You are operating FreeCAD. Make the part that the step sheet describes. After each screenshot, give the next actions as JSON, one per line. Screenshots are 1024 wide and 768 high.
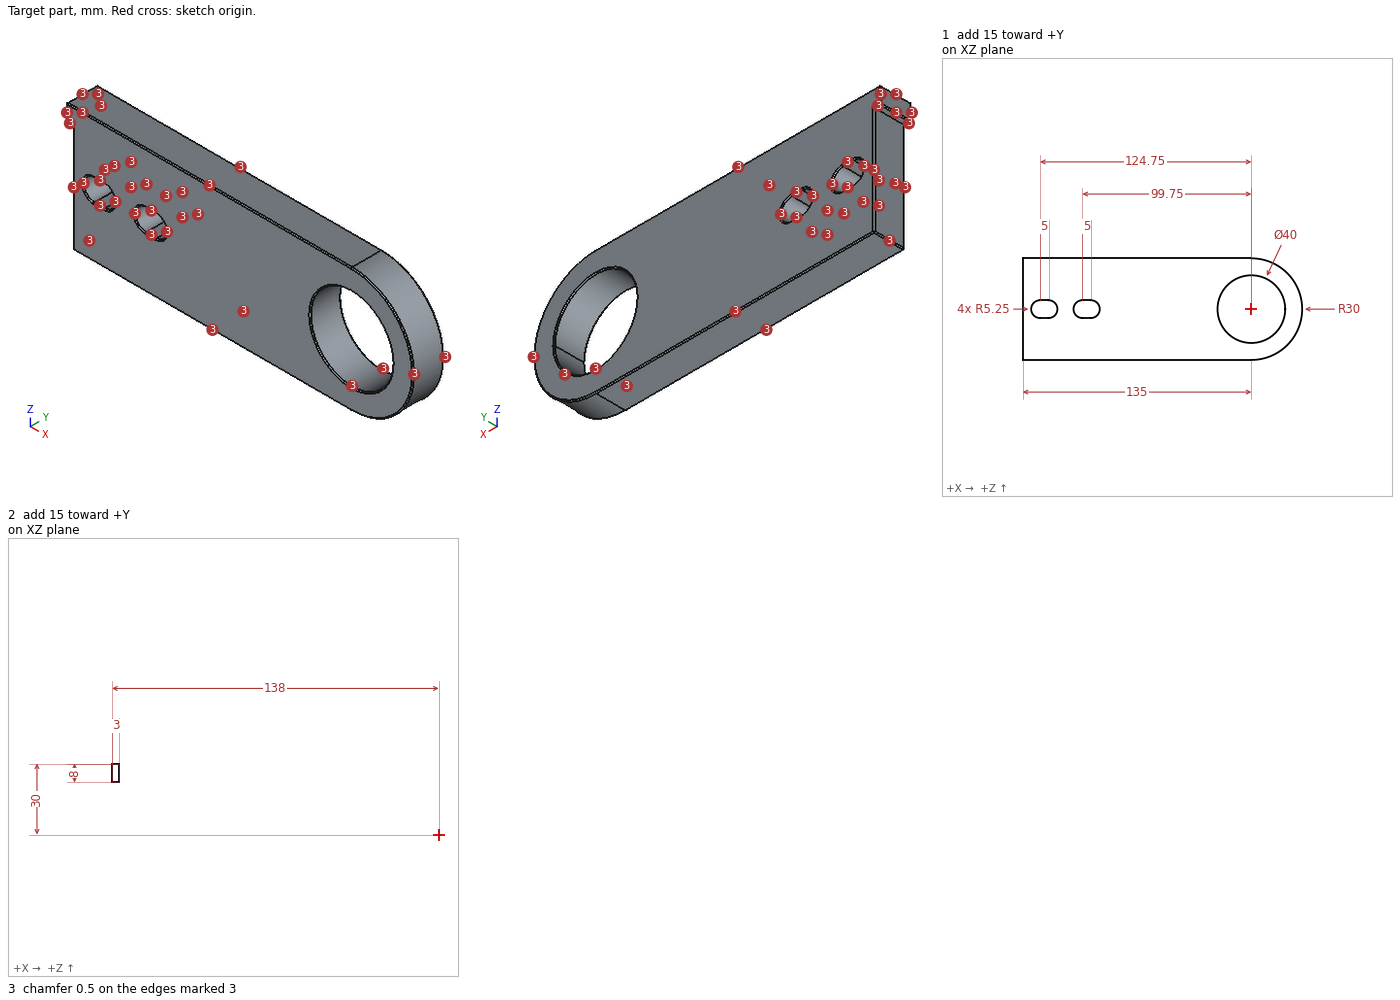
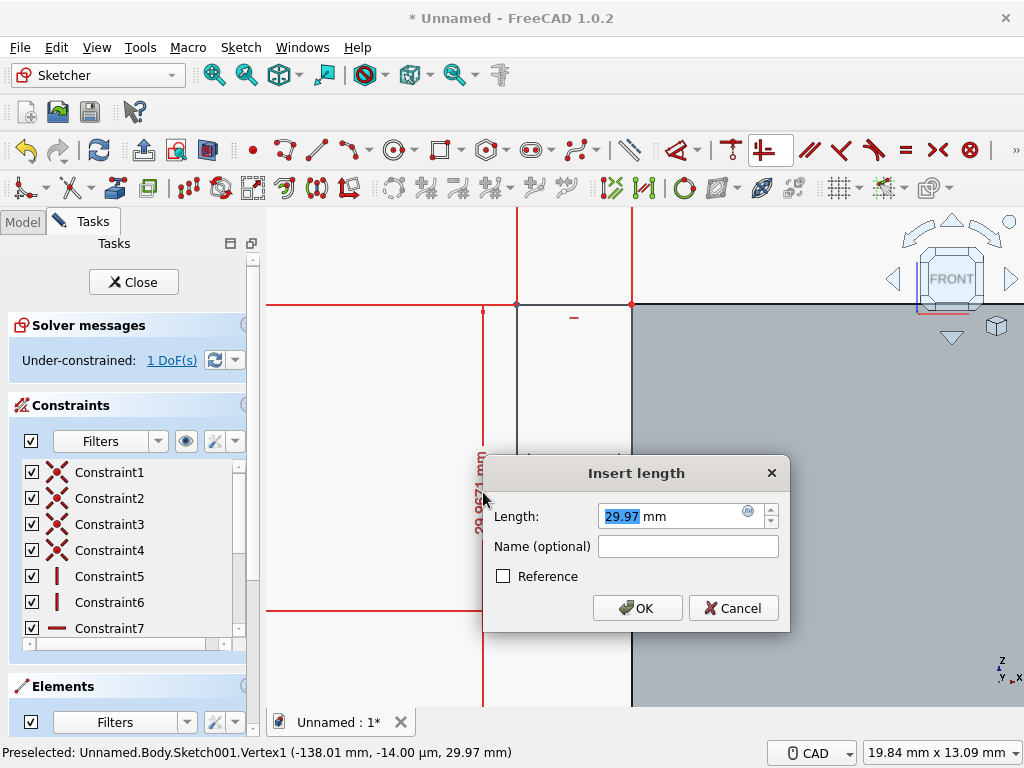
{"action": "type", "text": "30"}
{"action": "key", "text": "Return"}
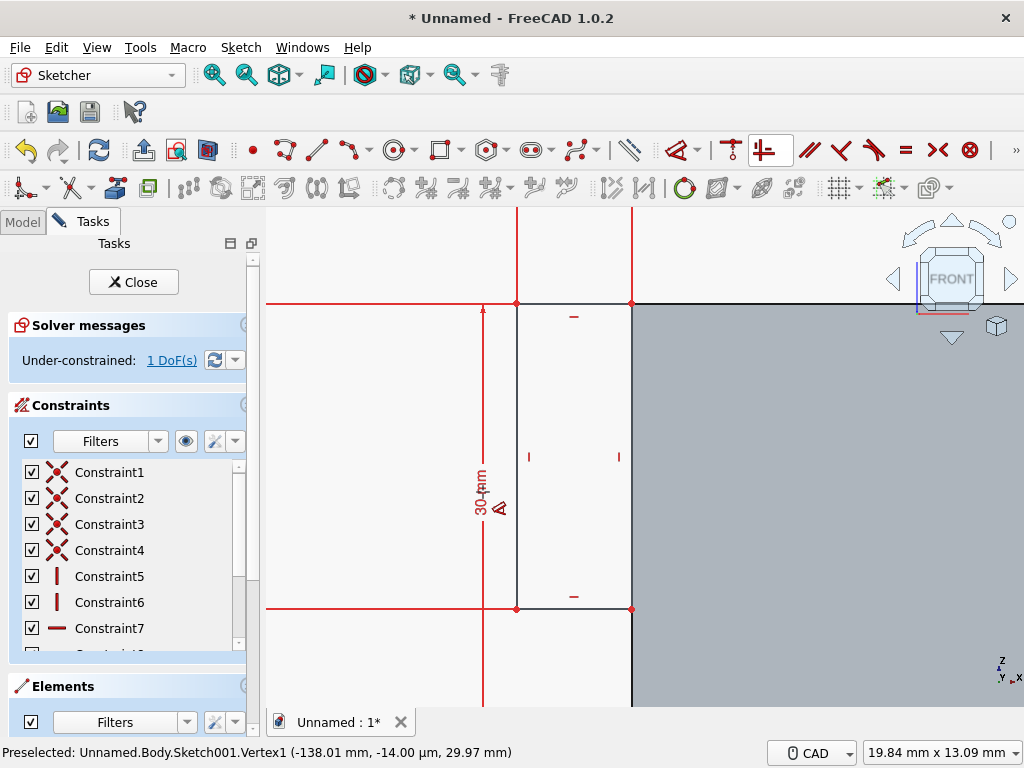
{"action": "left_click", "coordinate": [517, 304]}
{"action": "left_click", "coordinate": [688, 270]}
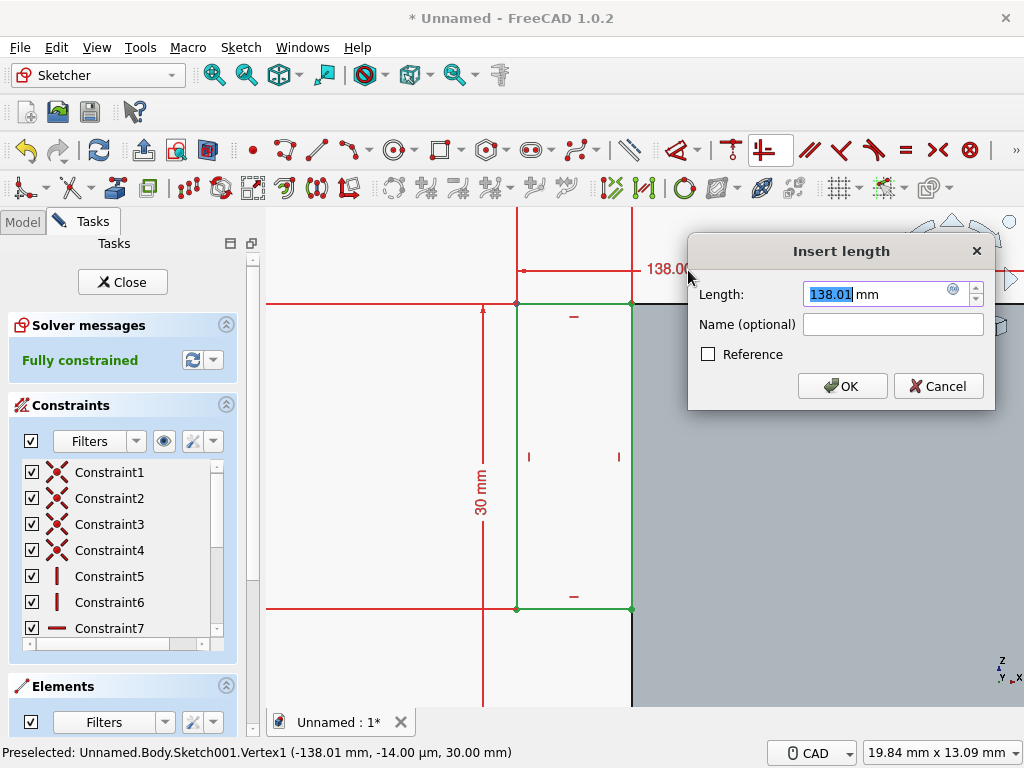
{"action": "type", "text": "138"}
{"action": "key", "text": "Return"}
{"action": "key", "text": "Escape"}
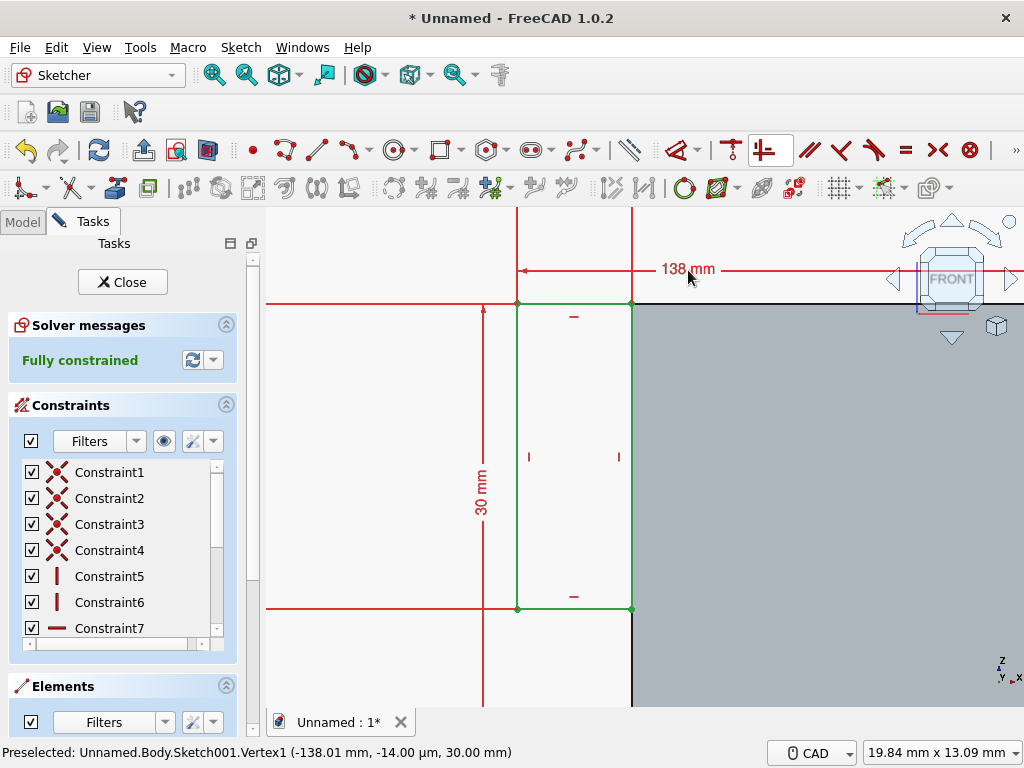
{"action": "left_click", "coordinate": [123, 282]}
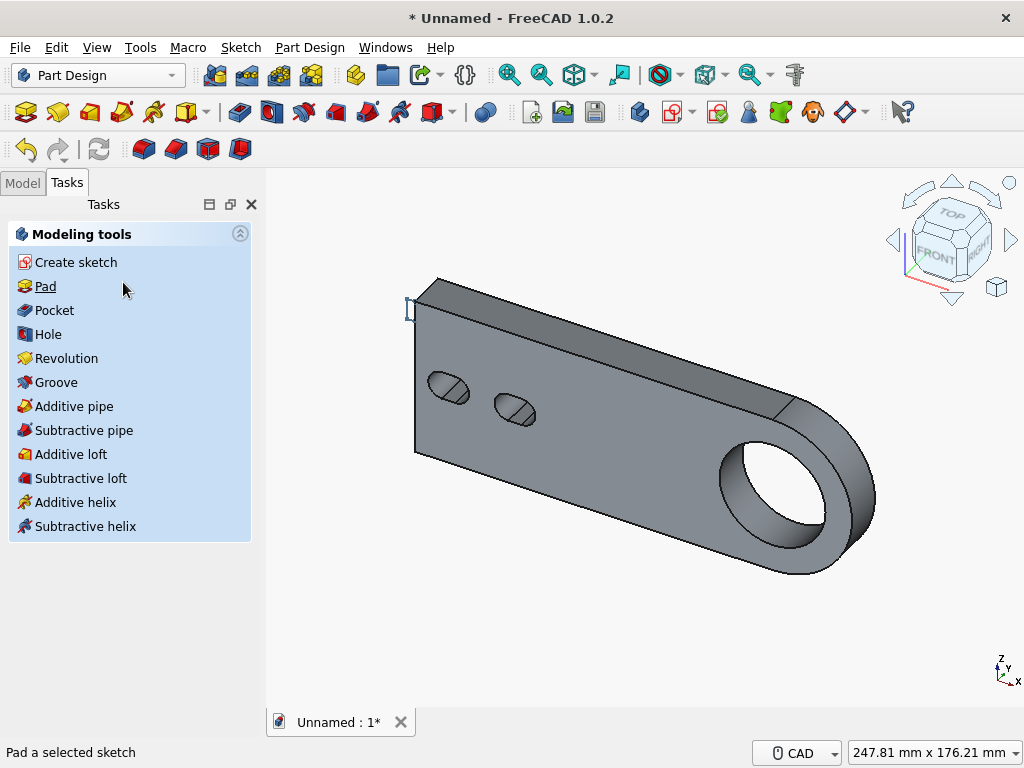
{"action": "left_click", "coordinate": [26, 112]}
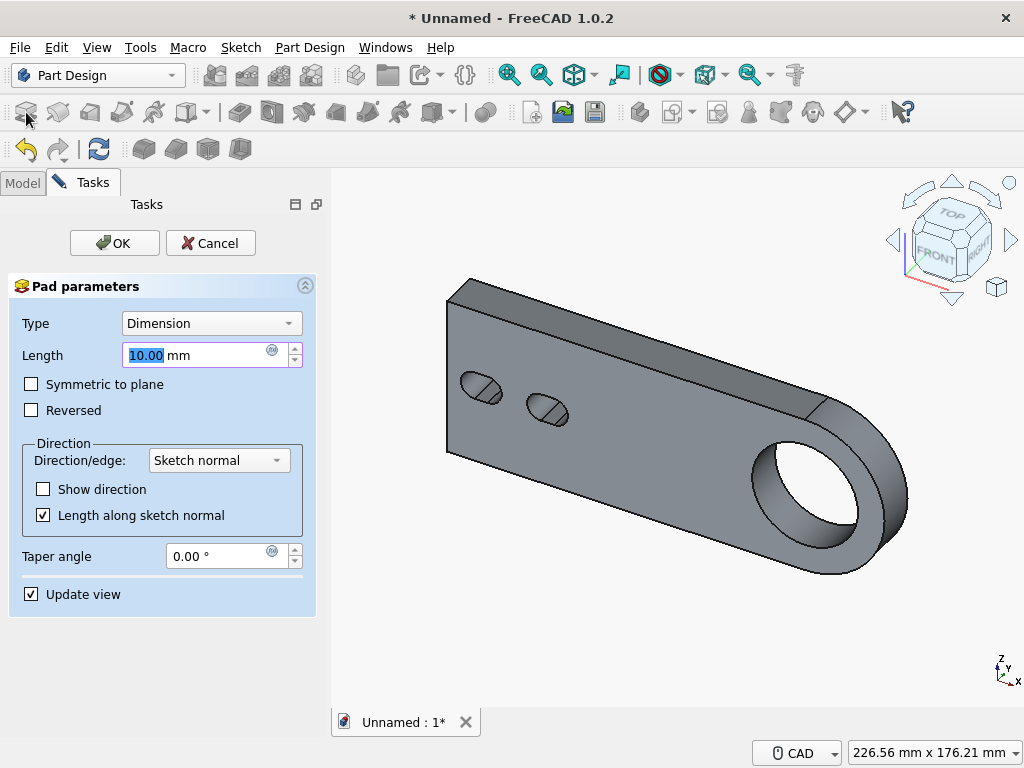
{"action": "type", "text": "15"}
{"action": "key", "text": "Tab"}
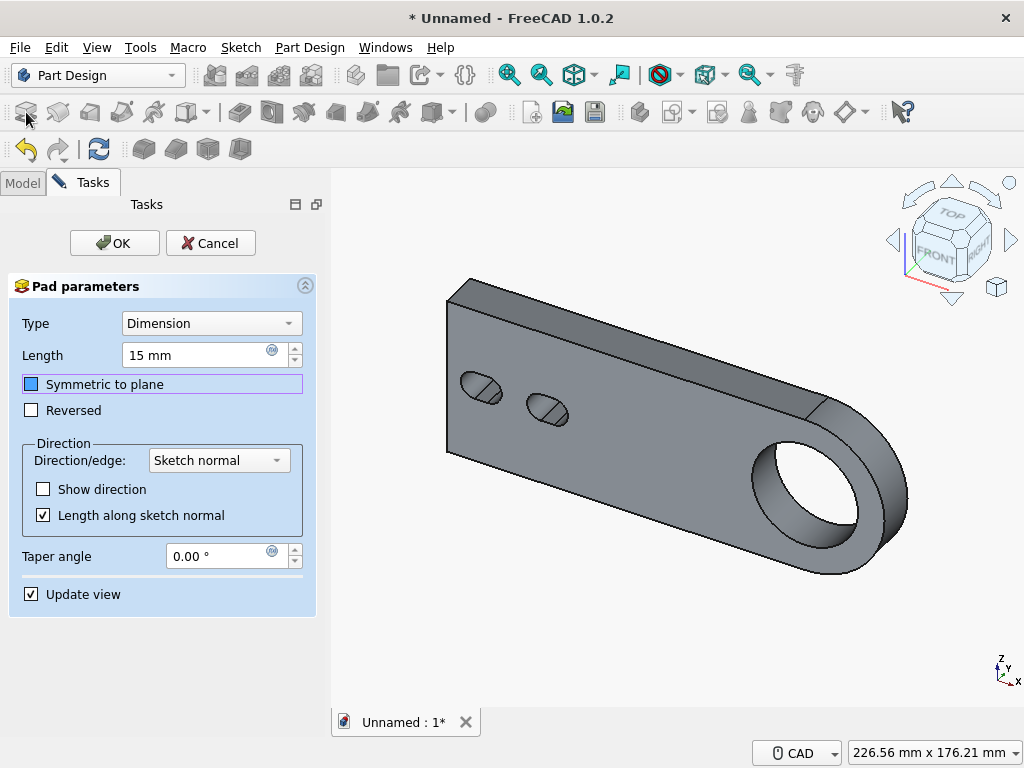
{"action": "left_click", "coordinate": [30, 410]}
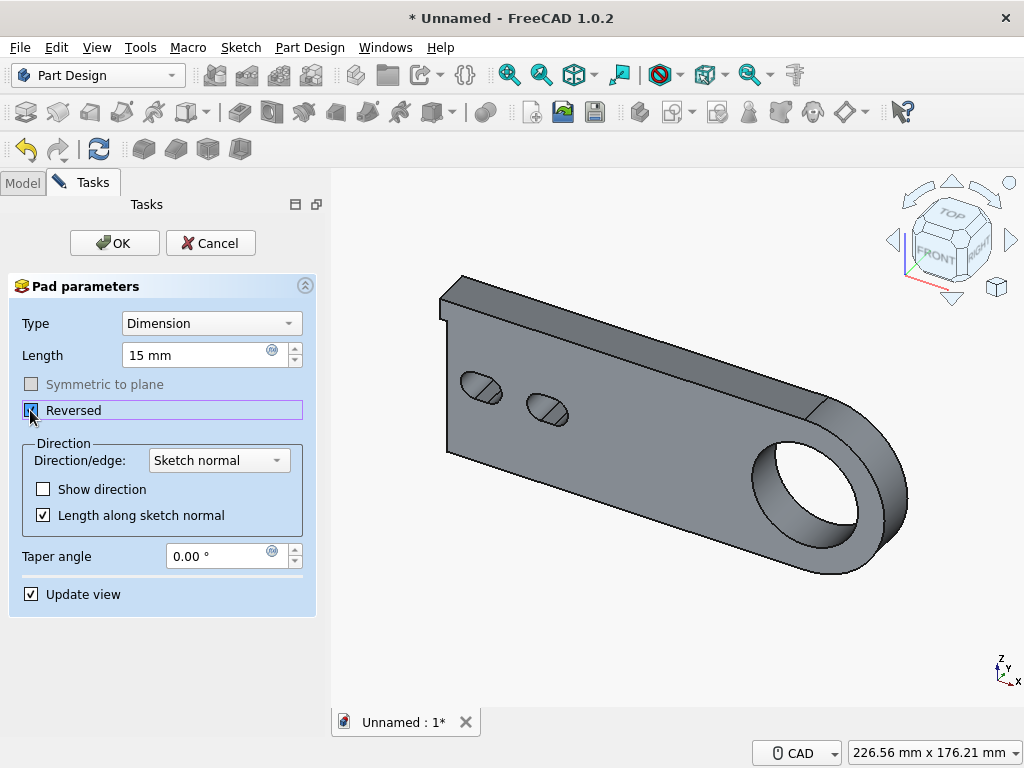
{"action": "left_click", "coordinate": [115, 243]}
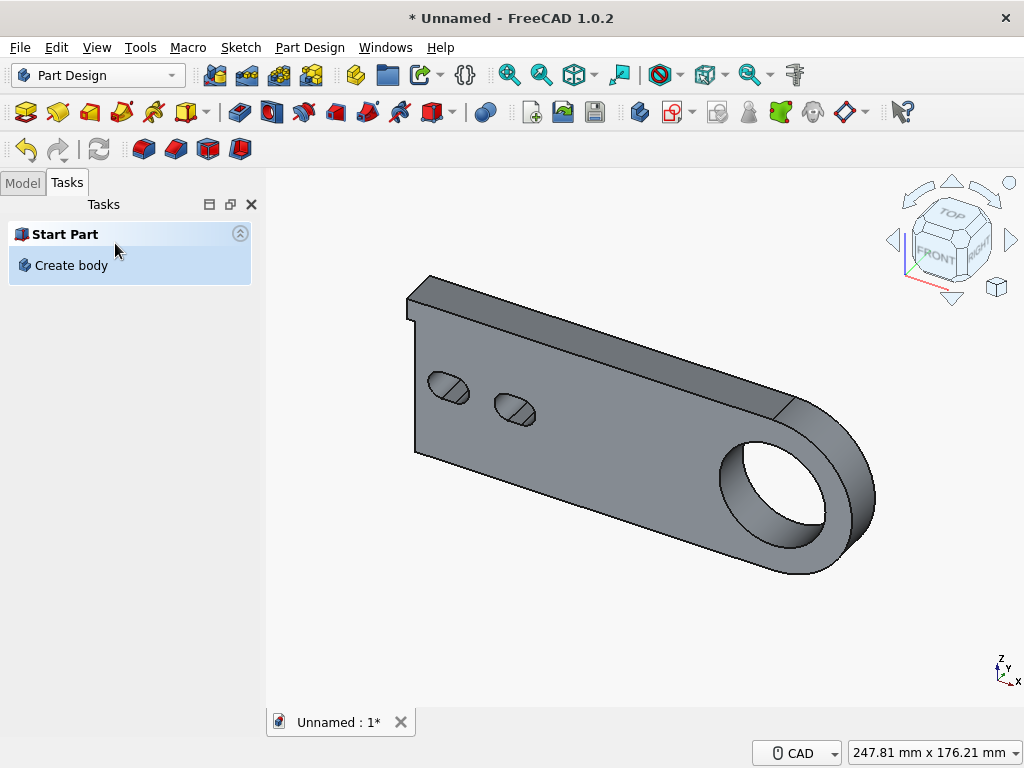
{"action": "left_click", "coordinate": [630, 447]}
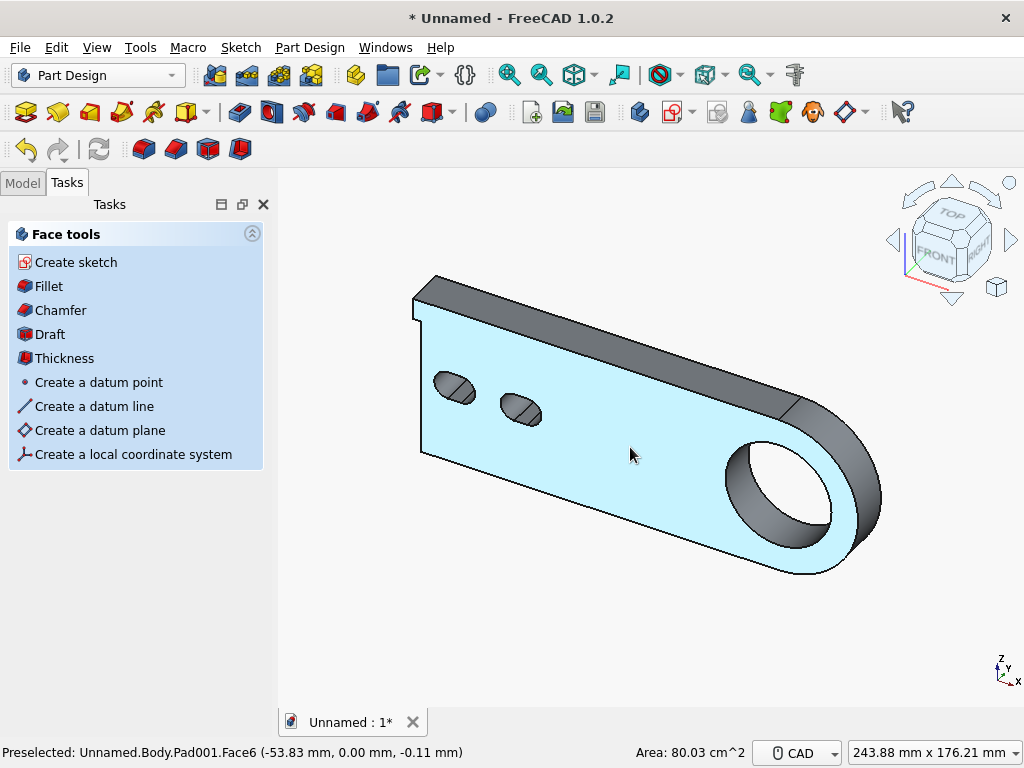
{"action": "key", "text": "0"}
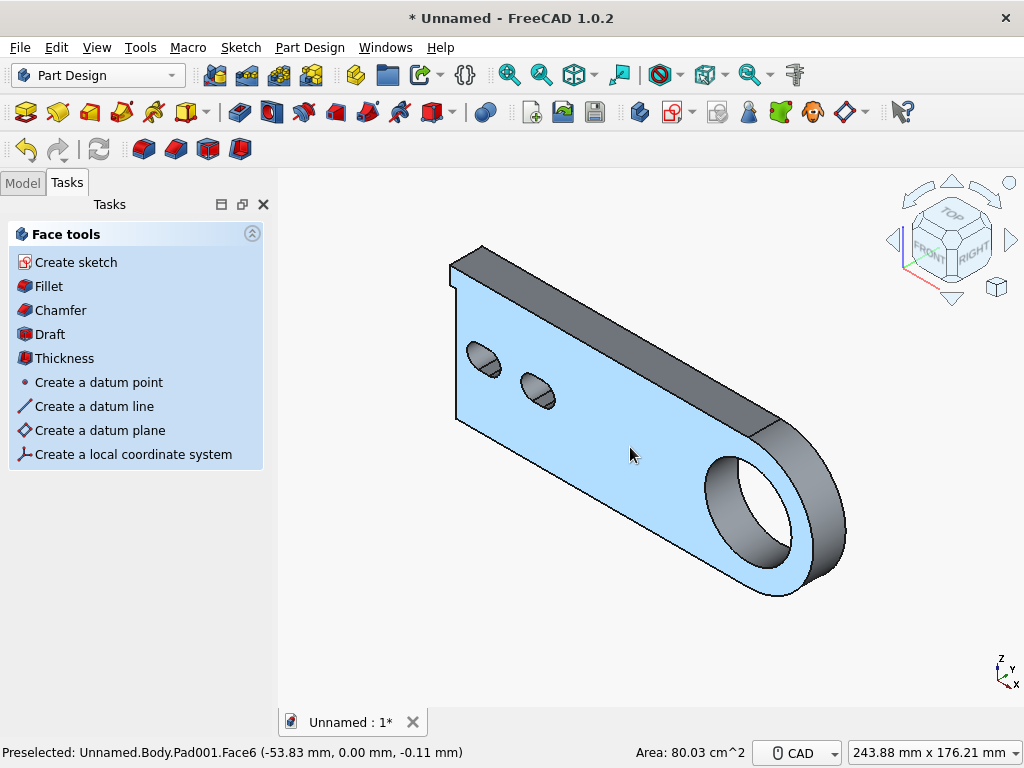
{"action": "key", "text": "2"}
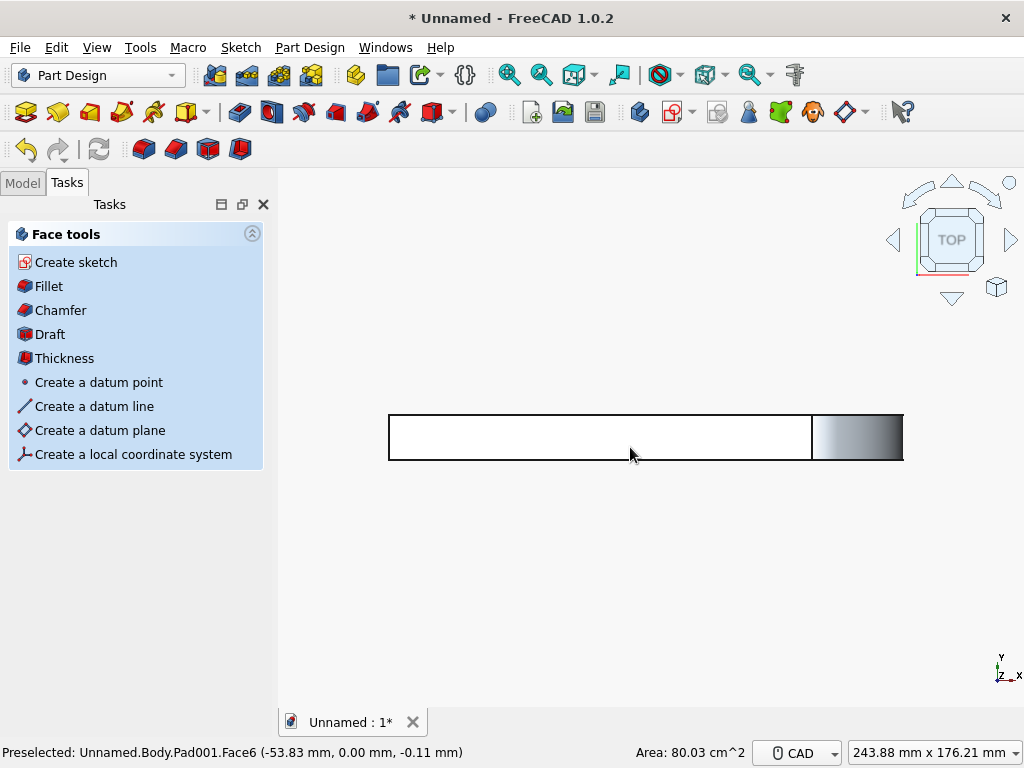
{"action": "left_click", "coordinate": [389, 436], "text": "ctrl"}